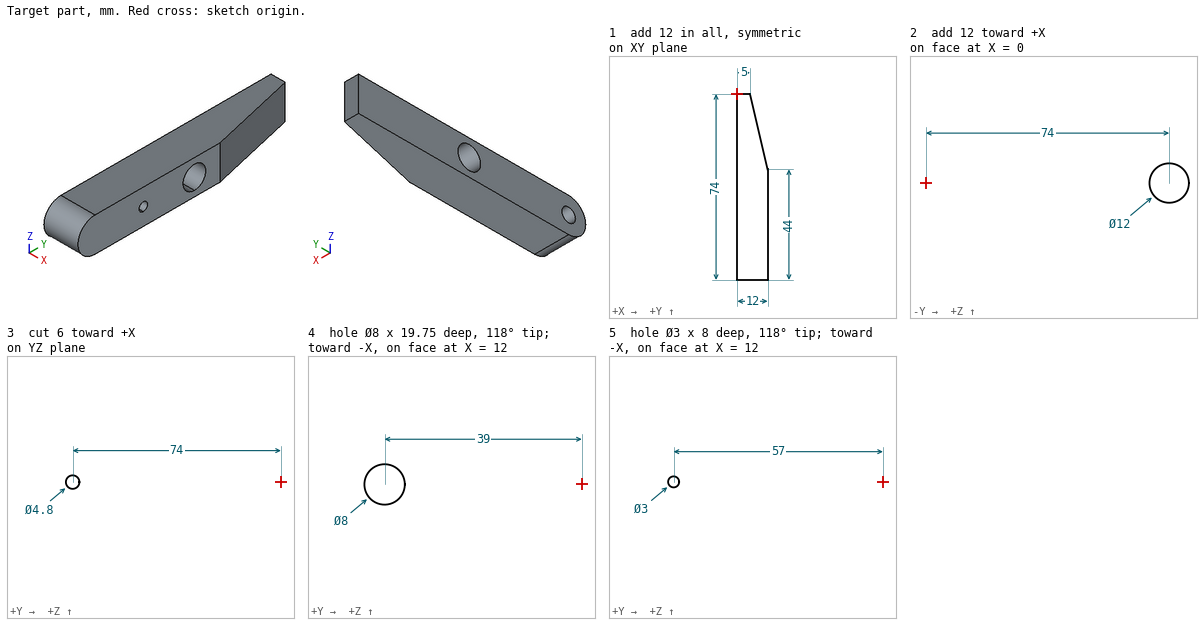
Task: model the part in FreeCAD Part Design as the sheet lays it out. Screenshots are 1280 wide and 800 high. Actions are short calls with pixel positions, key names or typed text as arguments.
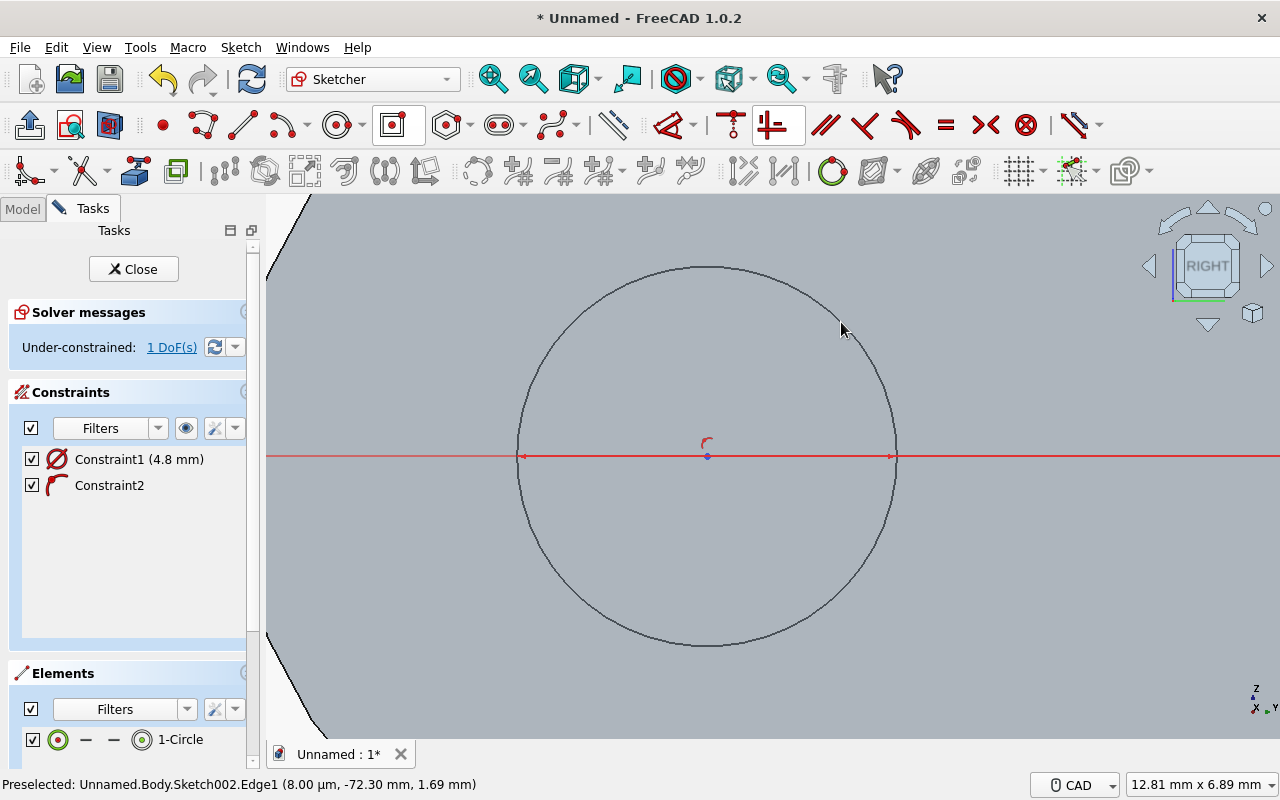
click(668, 126)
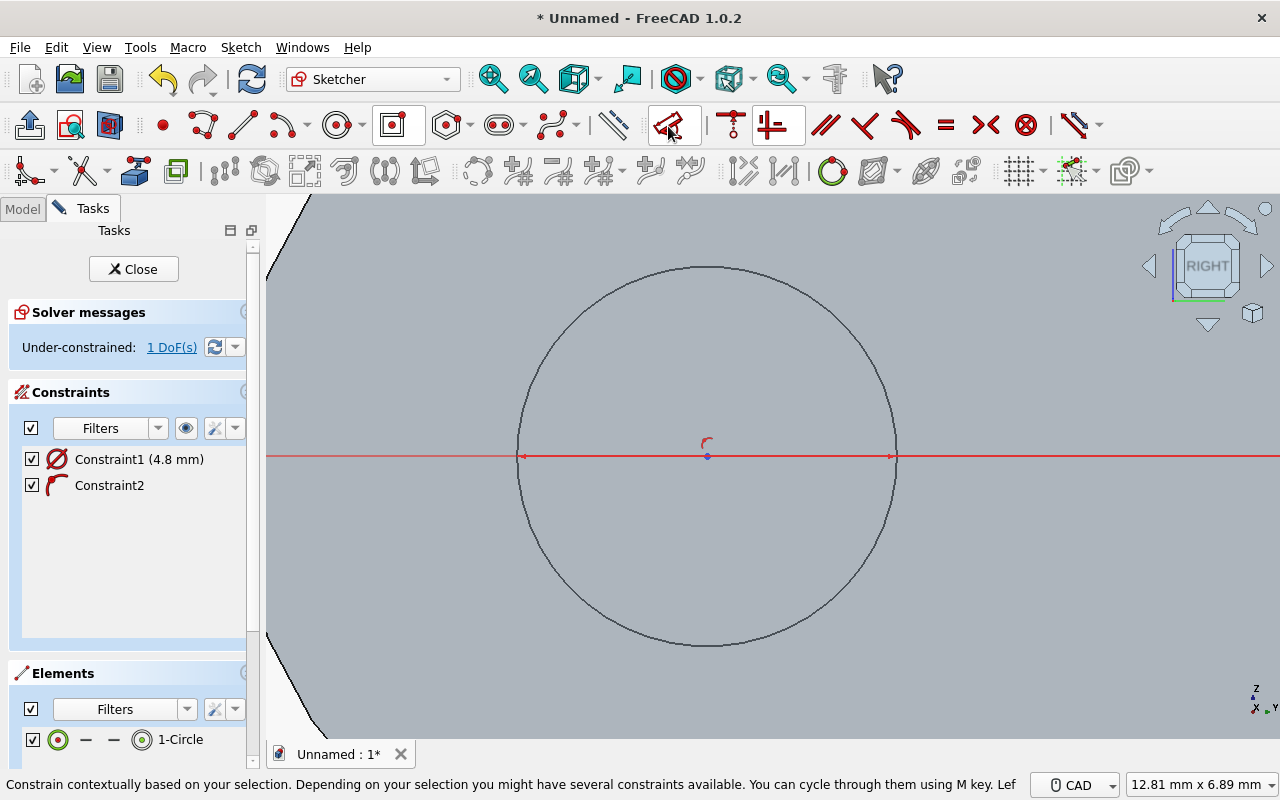
click(707, 456)
click(911, 490)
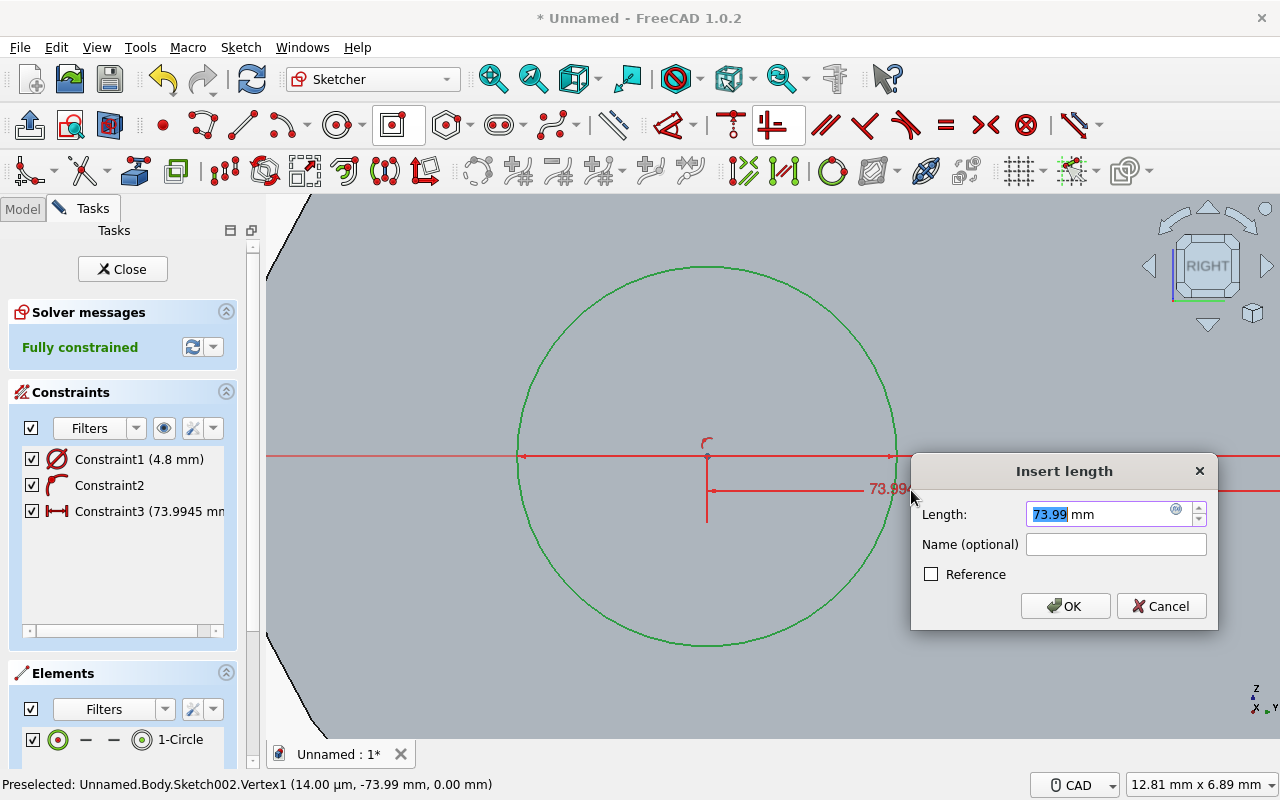
text(74)
key(Return)
key(Escape)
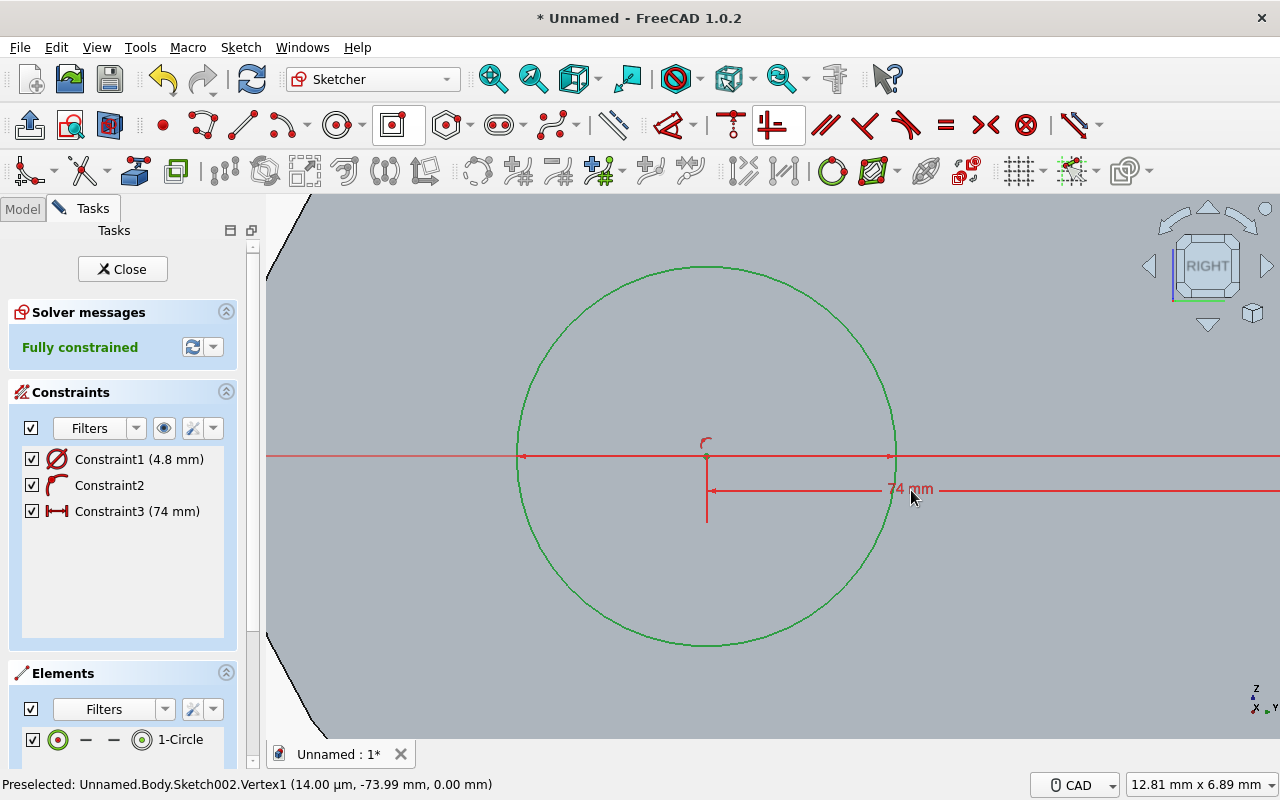
click(123, 269)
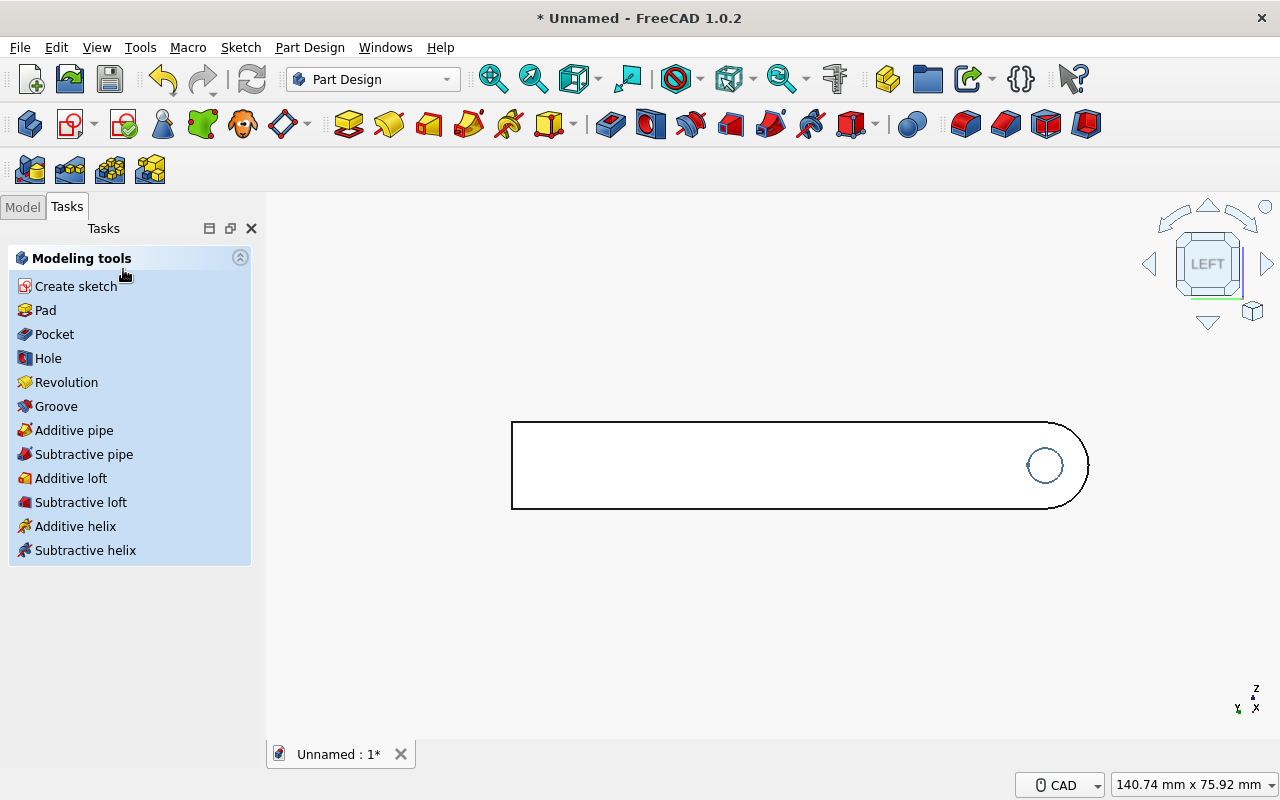
click(612, 124)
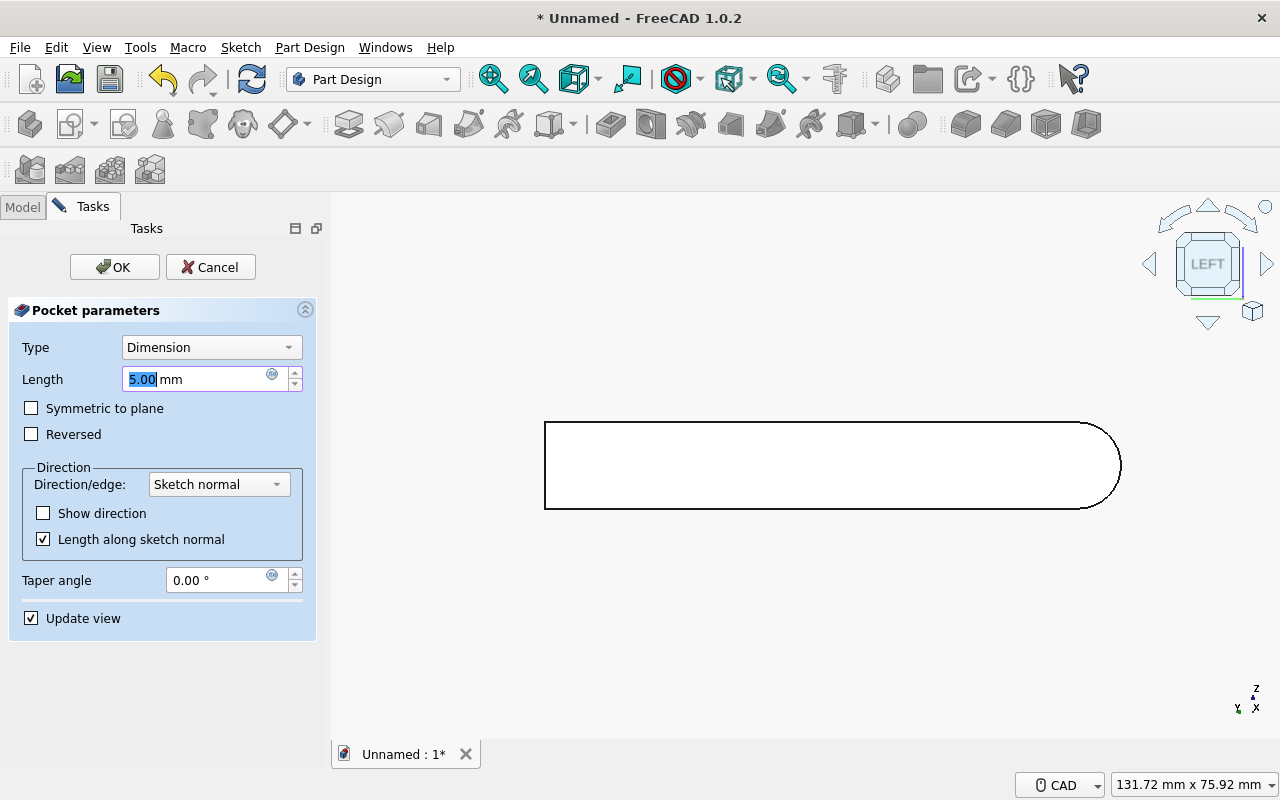
text(6)
key(Tab)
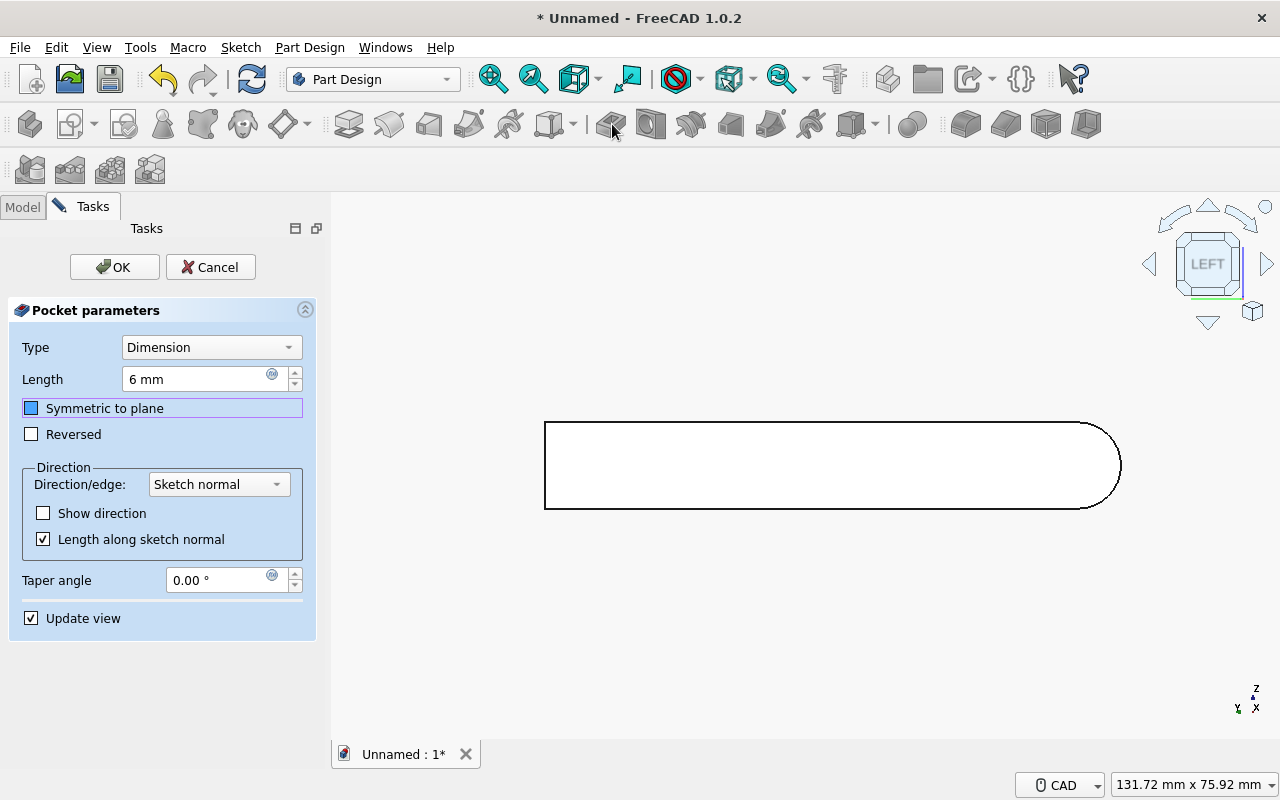
click(30, 434)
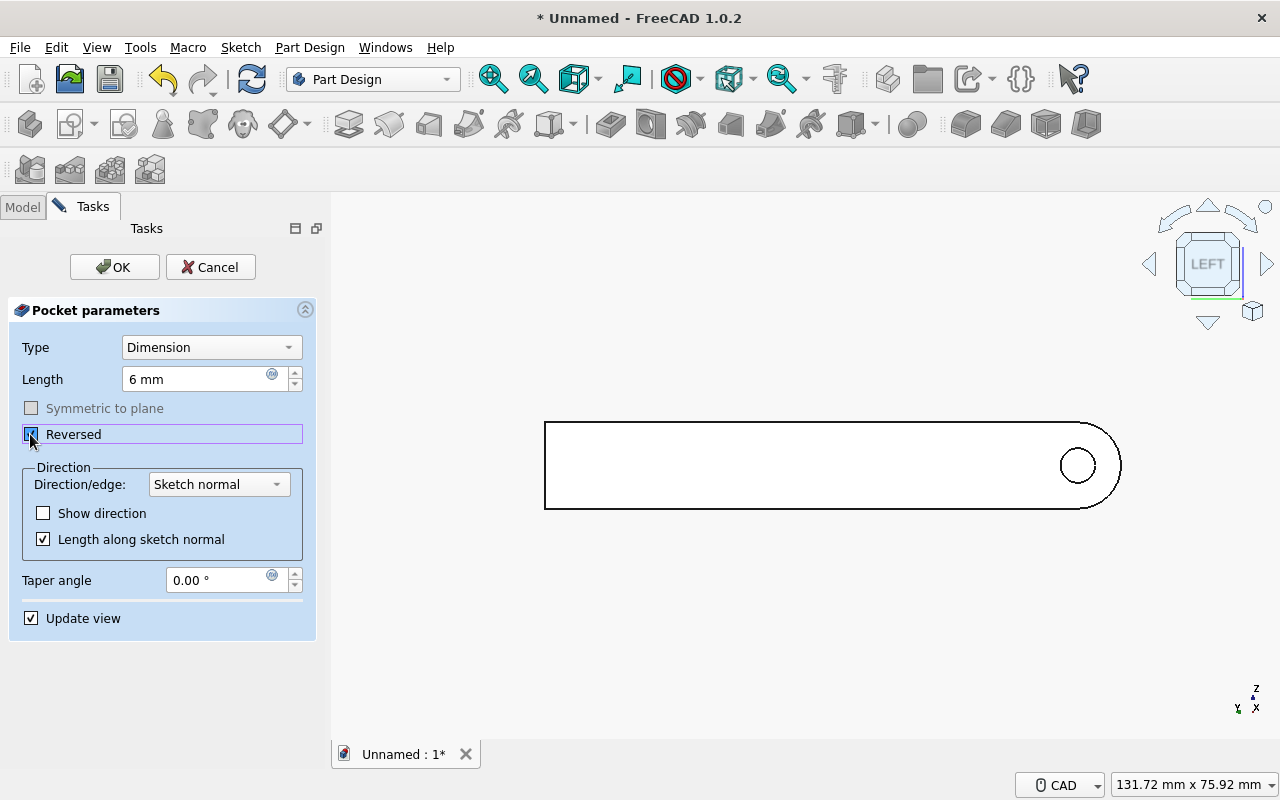
click(115, 267)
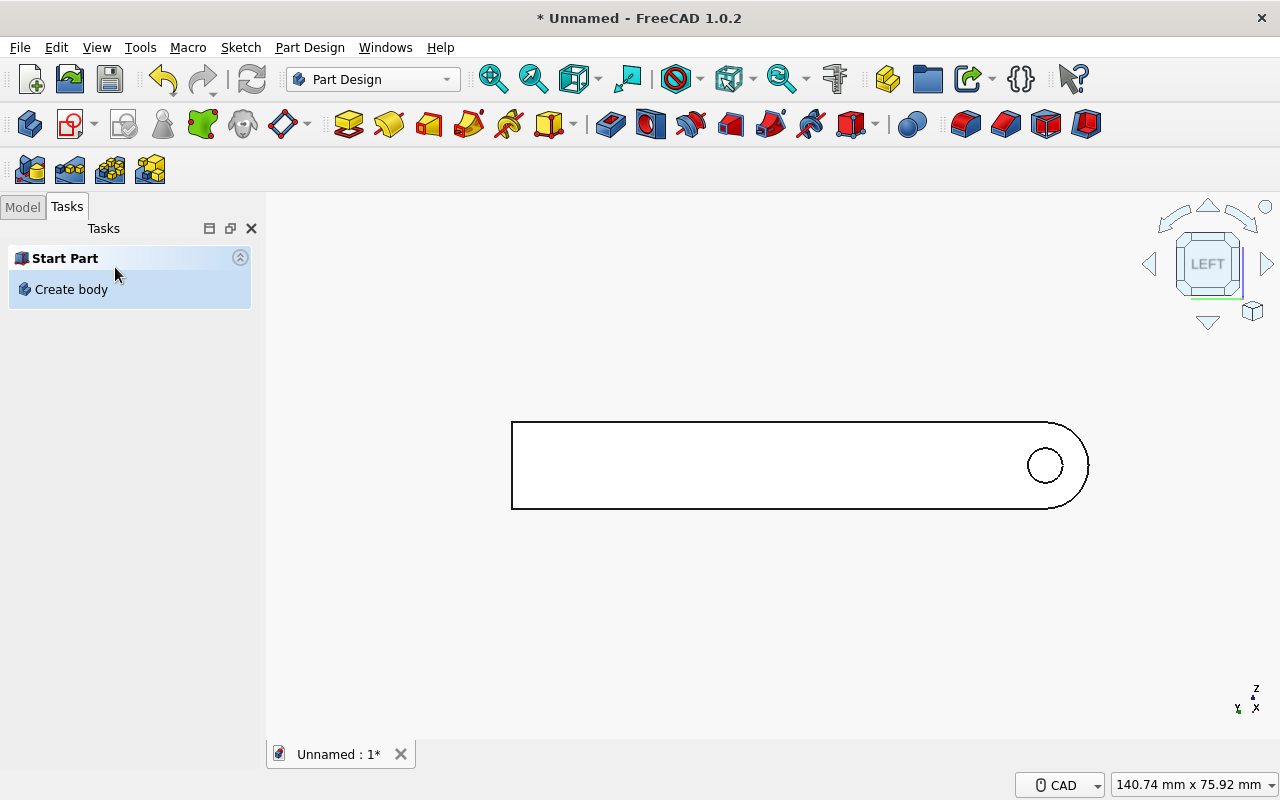
key(0)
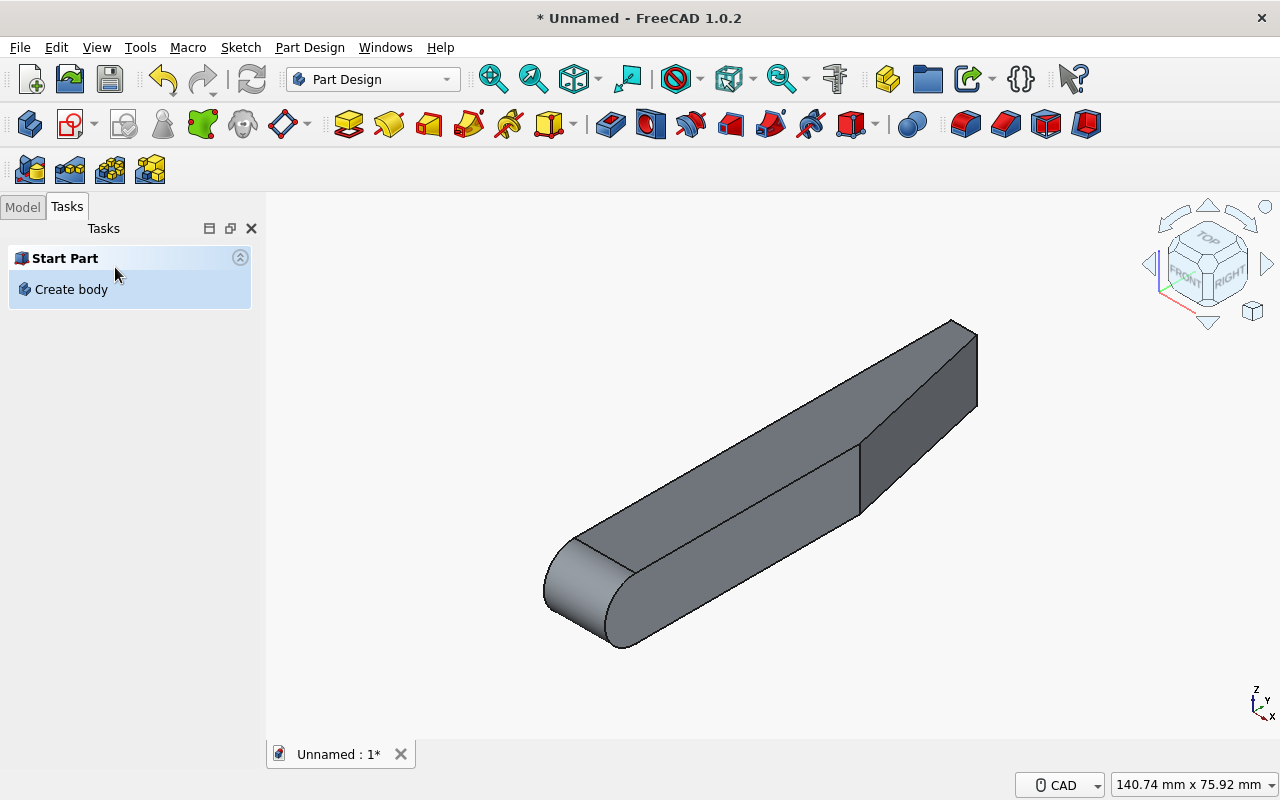
click(805, 510)